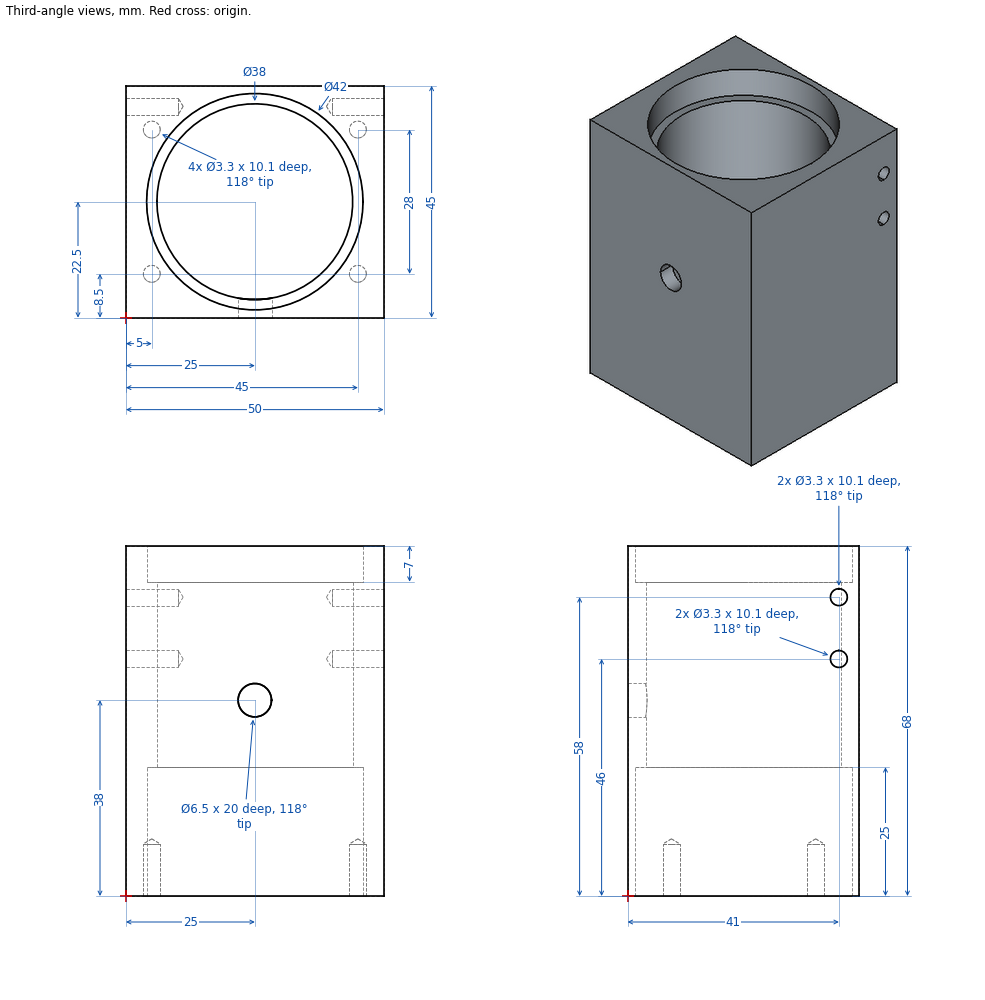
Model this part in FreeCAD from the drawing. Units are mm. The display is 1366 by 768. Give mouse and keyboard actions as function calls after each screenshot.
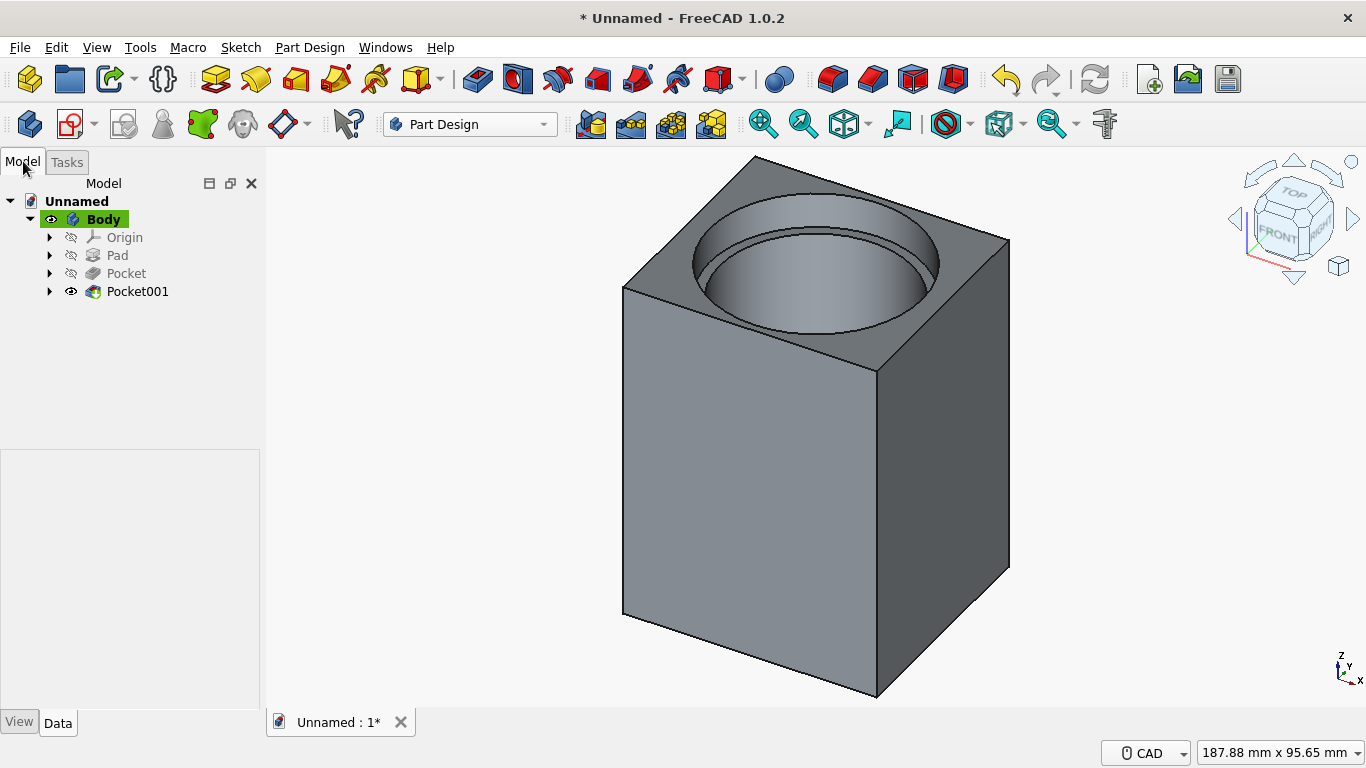
click(50, 237)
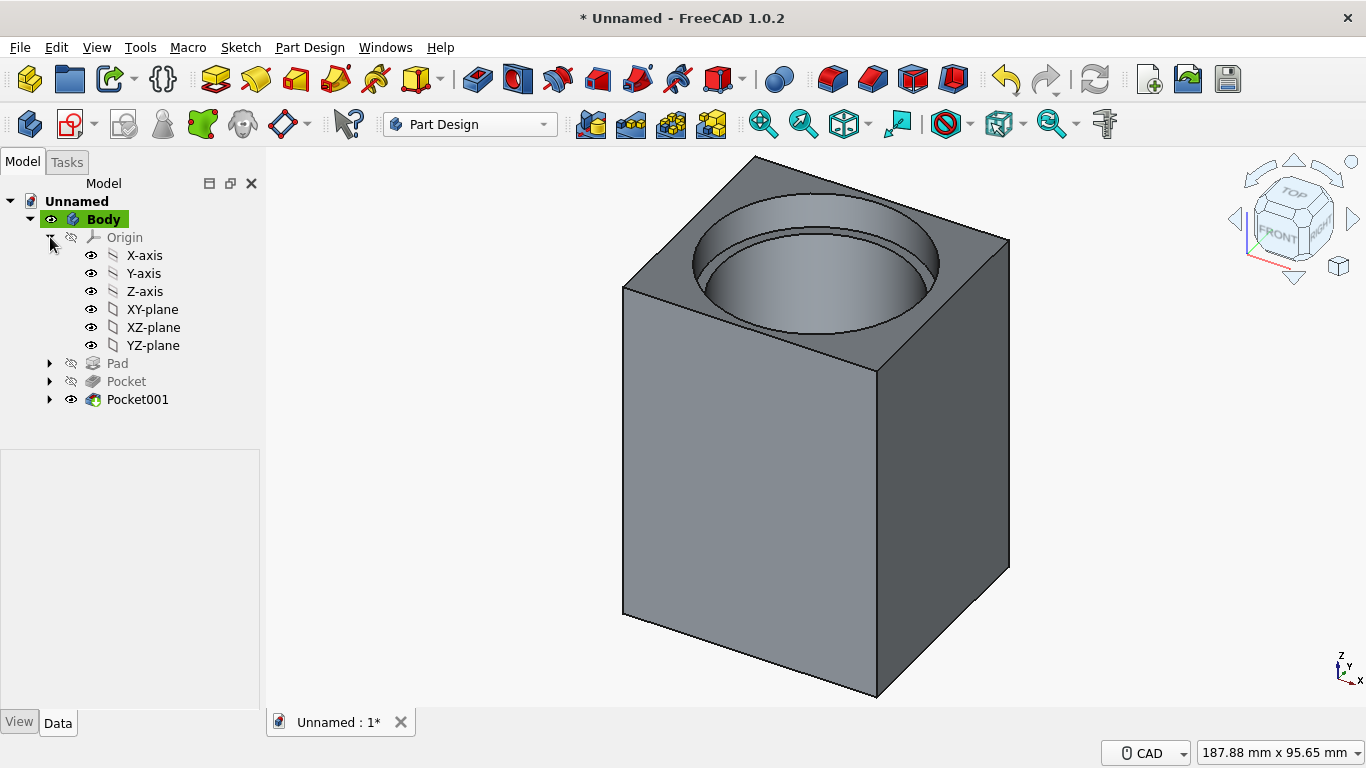
click(136, 309)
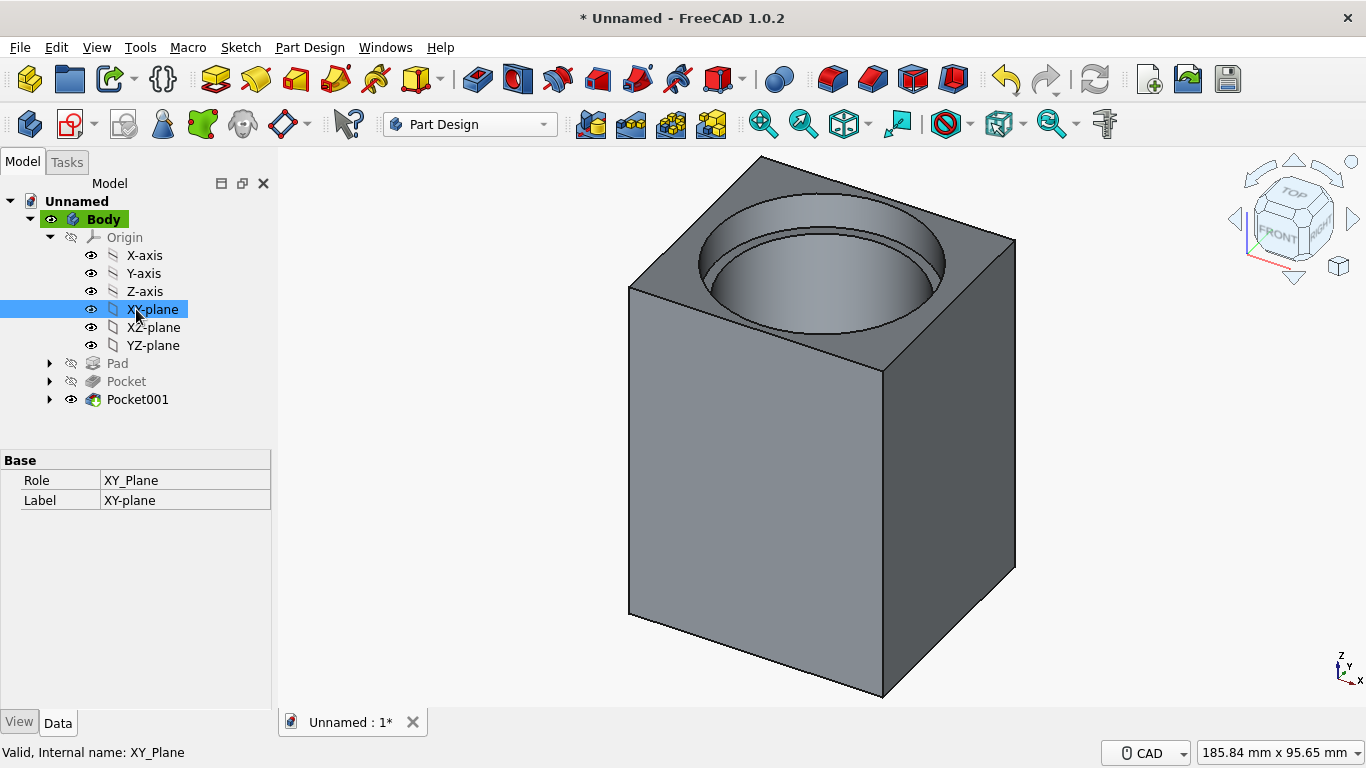
click(284, 124)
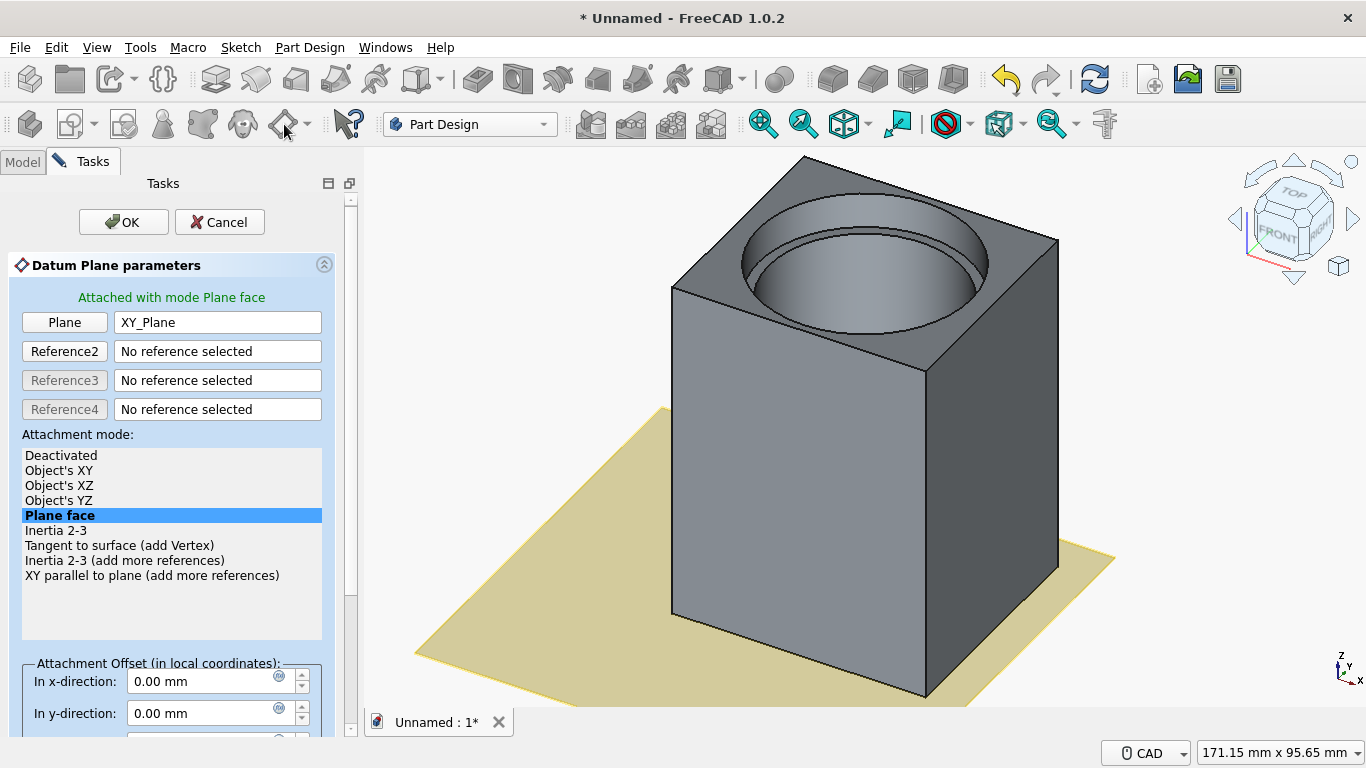
scroll(351, 464, down, 2)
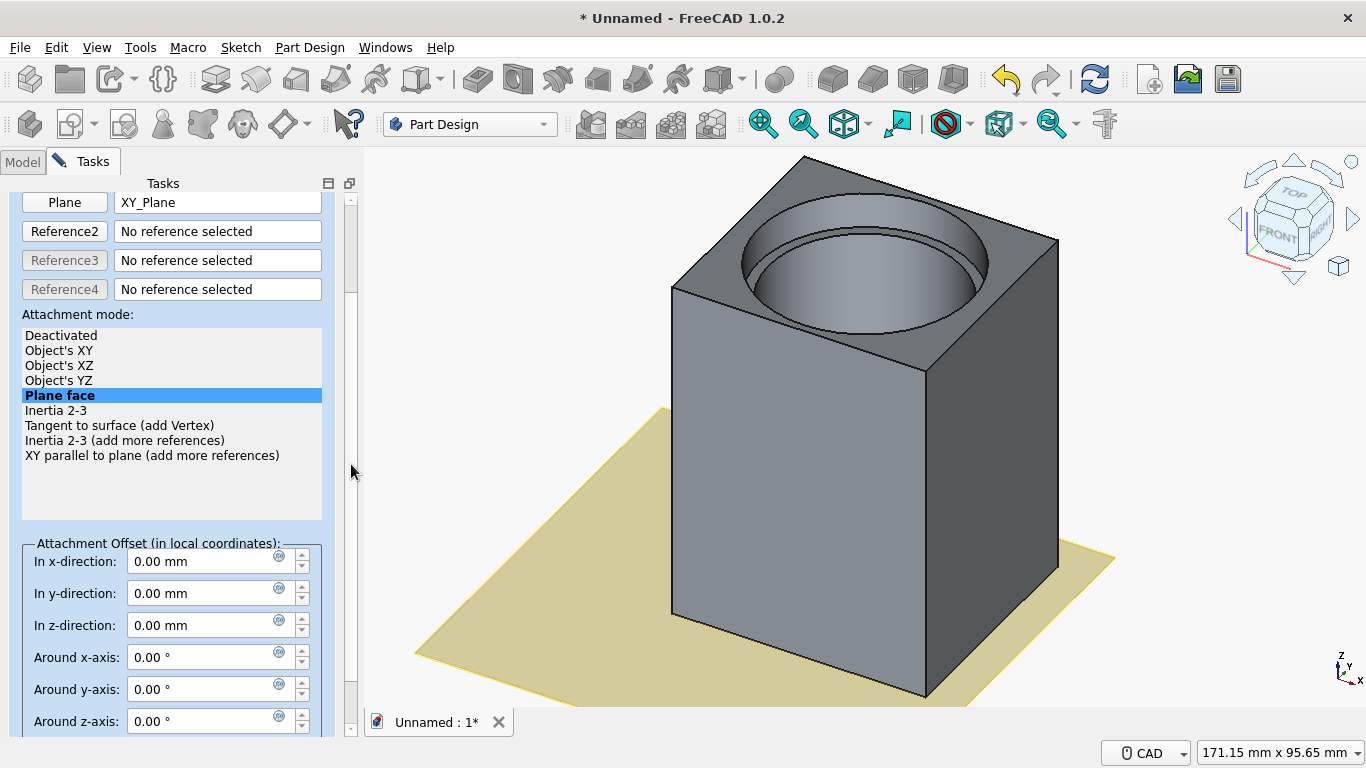
triple_click(210, 625)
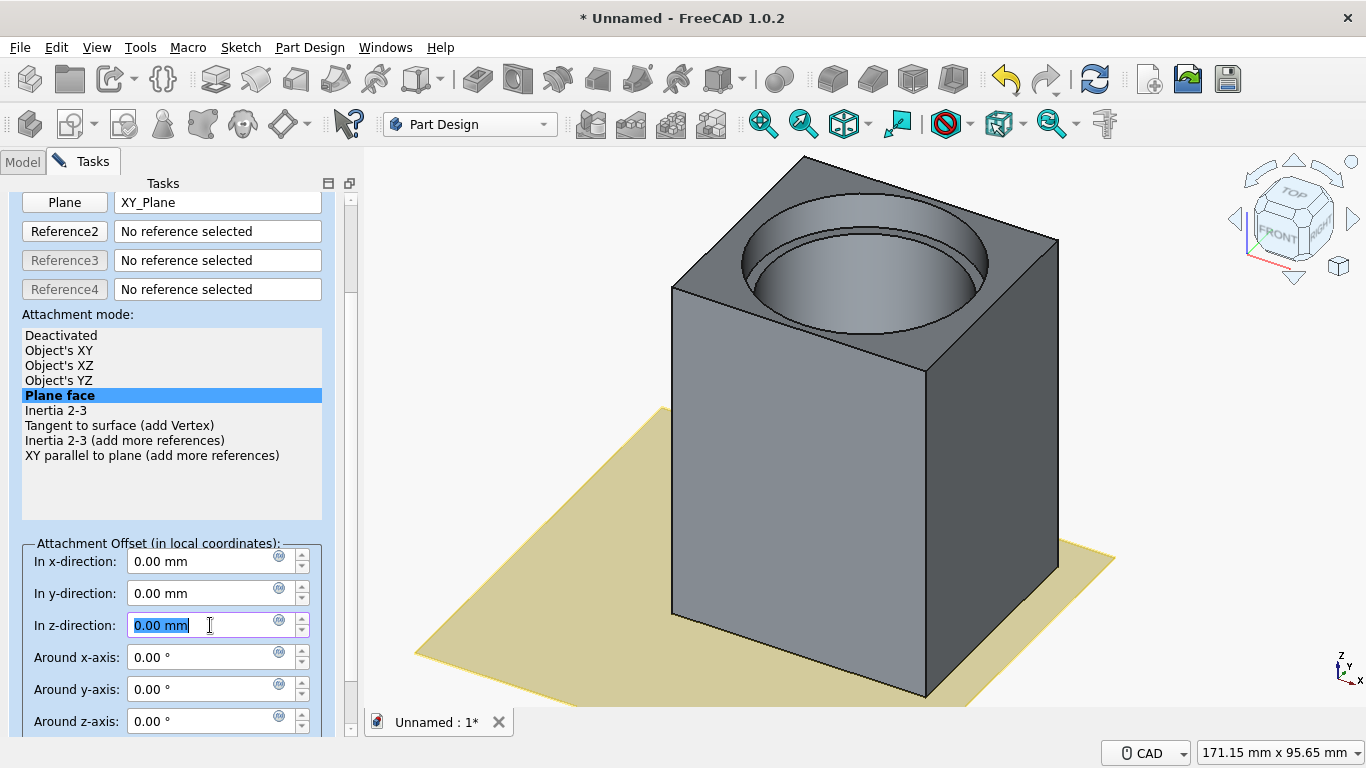
text(25)
key(Tab)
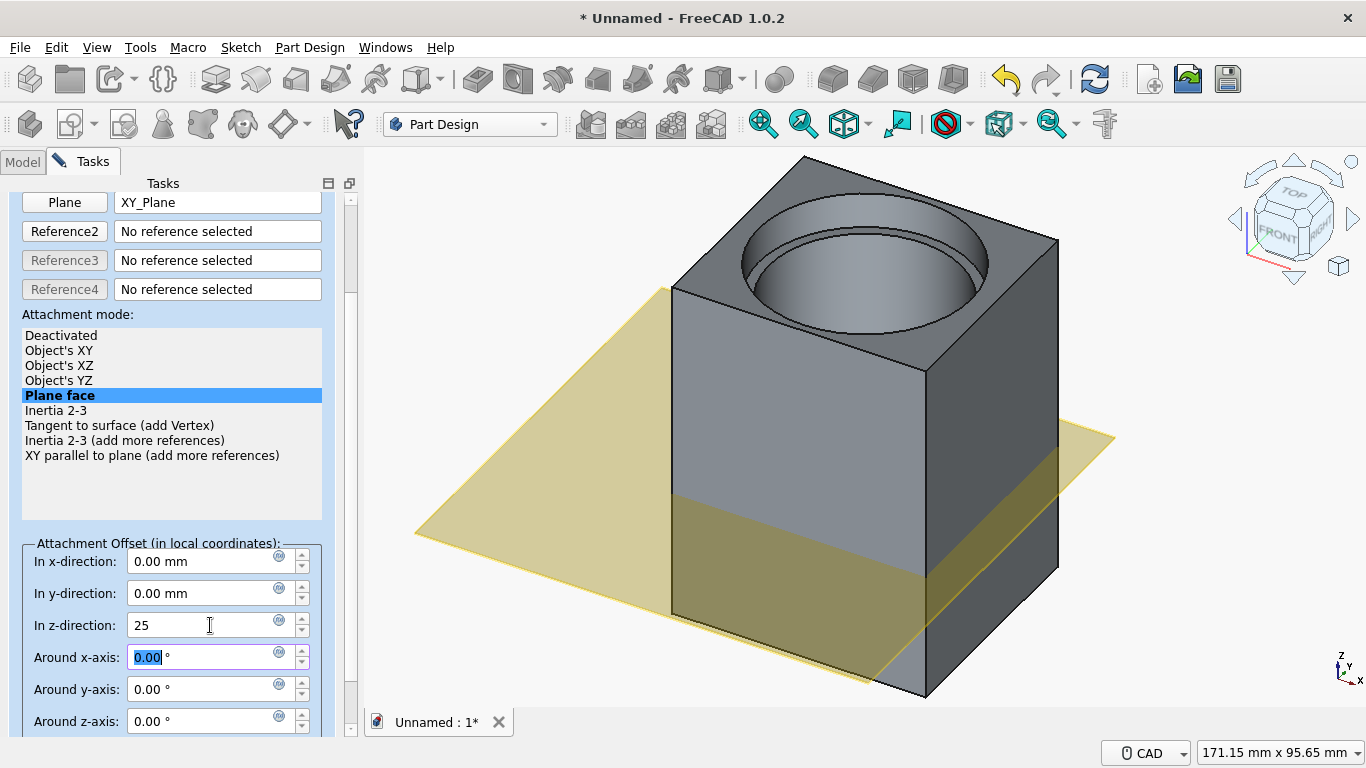
scroll(351, 464, up, 3)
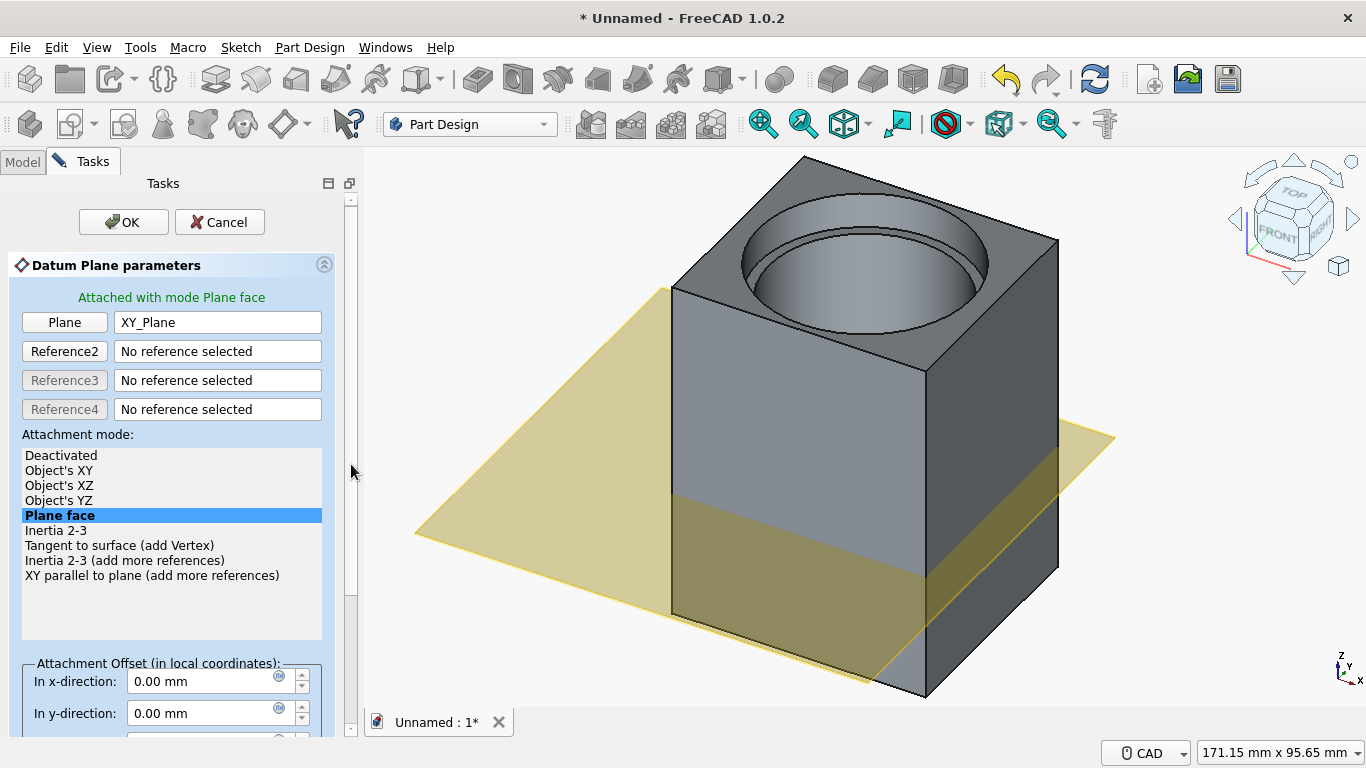
click(124, 222)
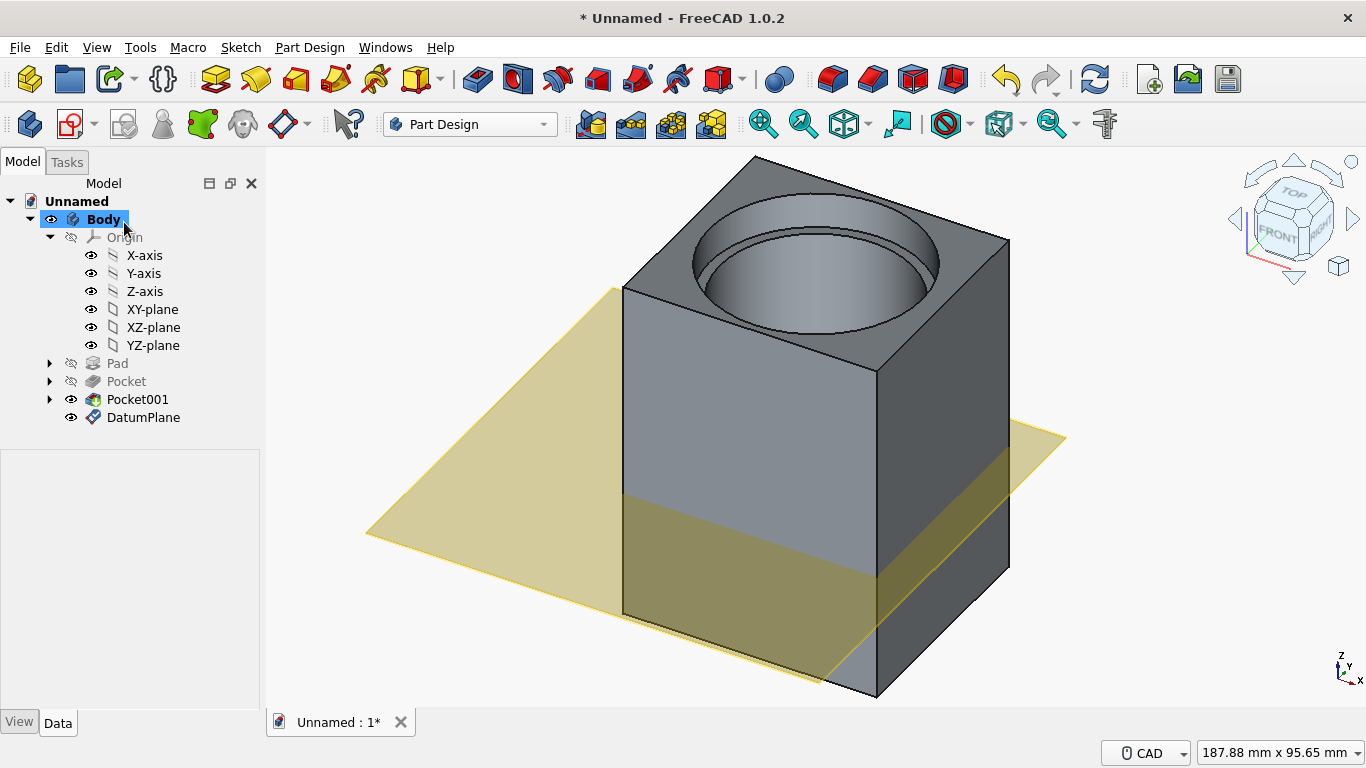
click(116, 417)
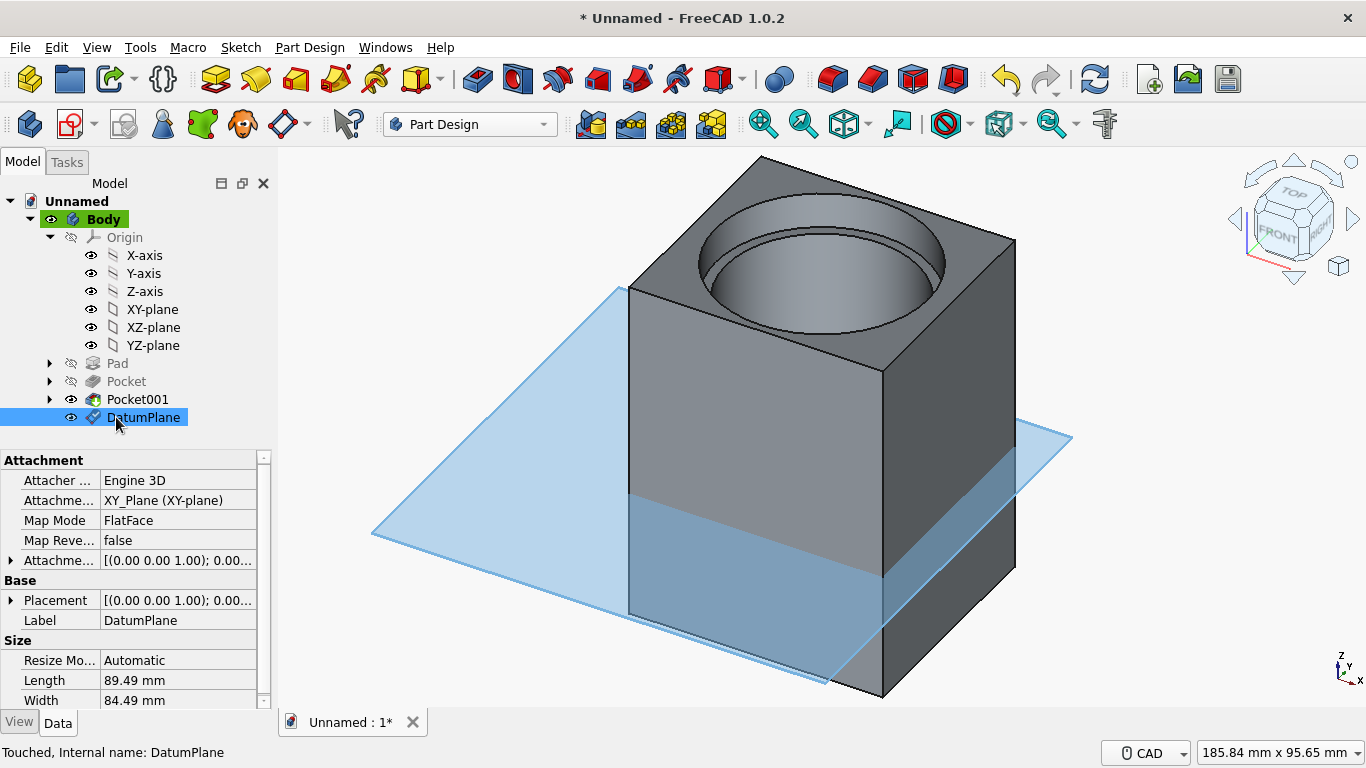
click(70, 124)